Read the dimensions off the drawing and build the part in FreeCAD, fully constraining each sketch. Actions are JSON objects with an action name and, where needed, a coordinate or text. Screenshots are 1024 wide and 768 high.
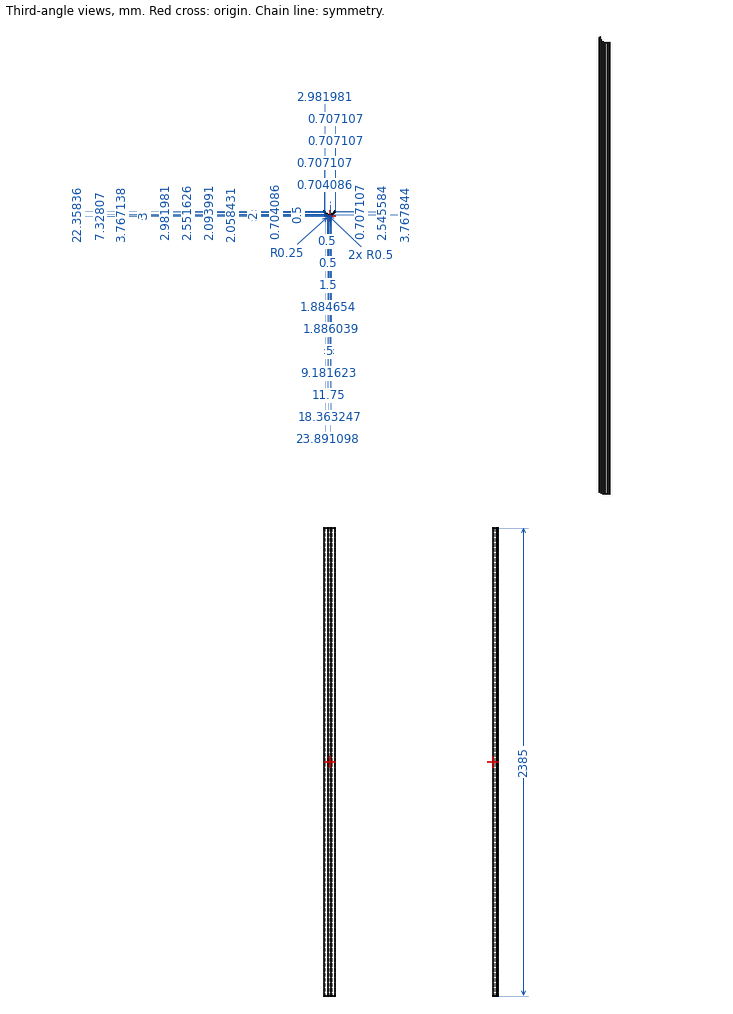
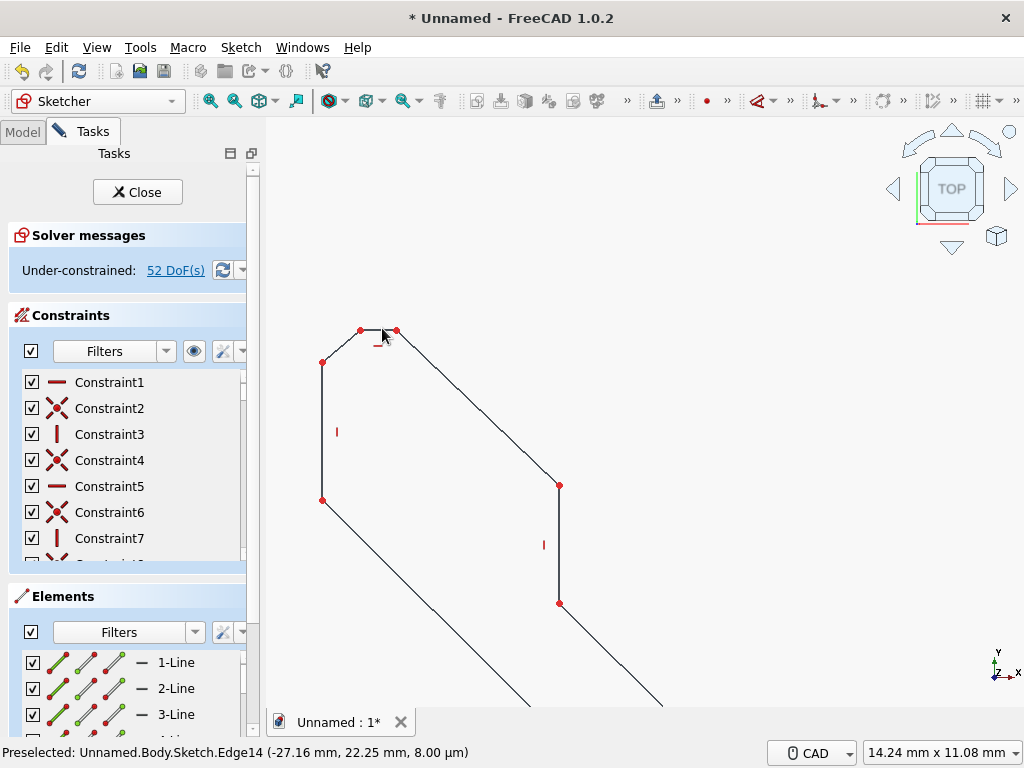
{"action": "scroll", "coordinate": [381, 333], "scroll_direction": "down", "scroll_amount": 10}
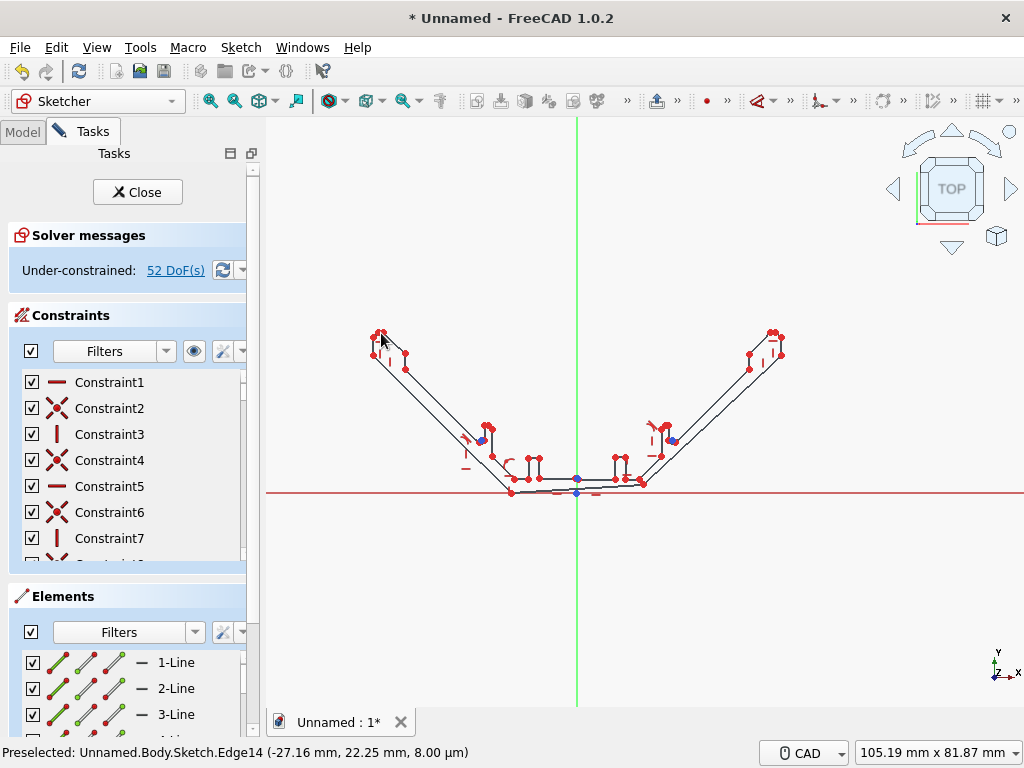
{"action": "scroll", "coordinate": [551, 491], "scroll_direction": "up", "scroll_amount": 9}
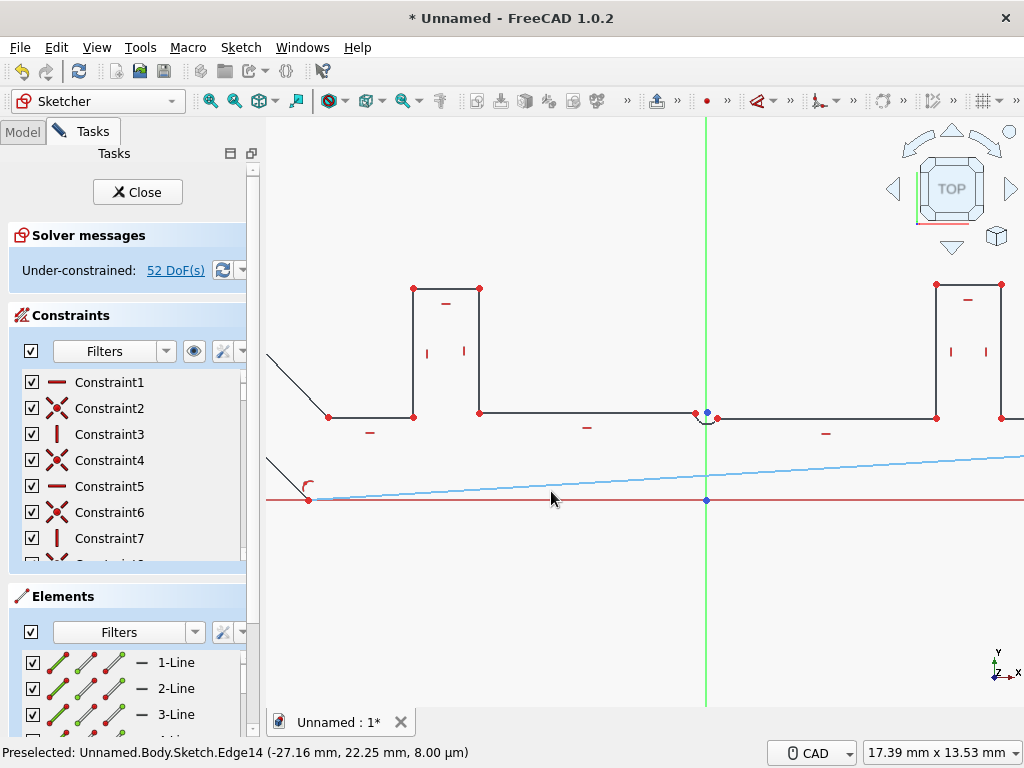
{"action": "left_click", "coordinate": [548, 485]}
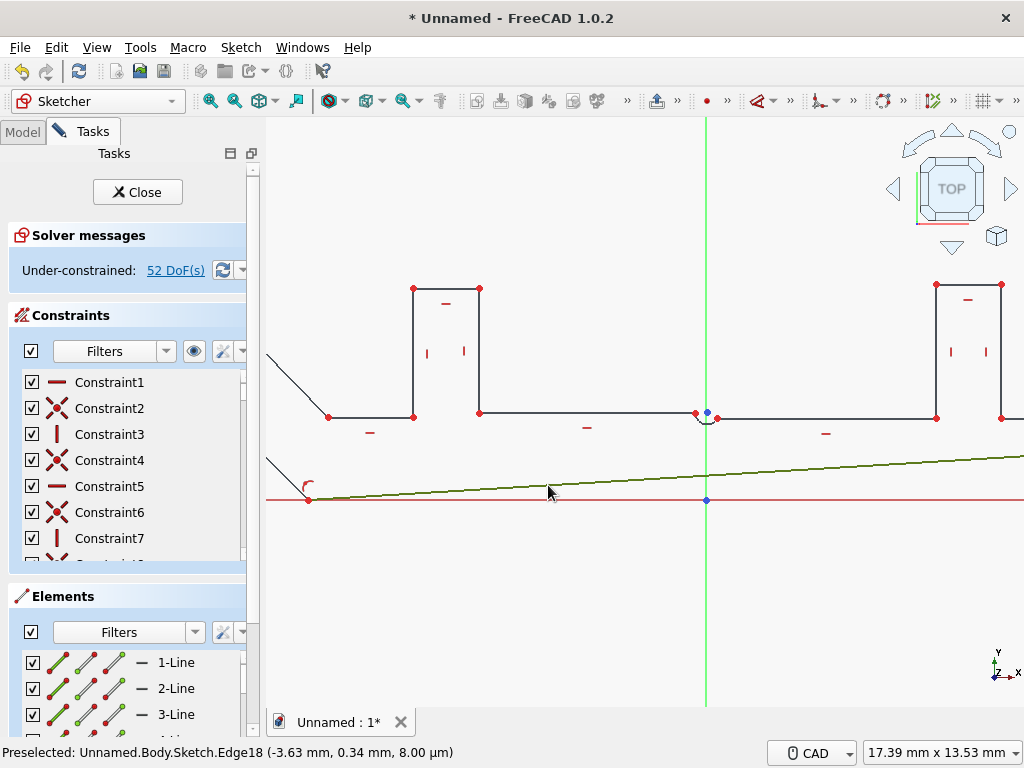
{"action": "key", "text": "h"}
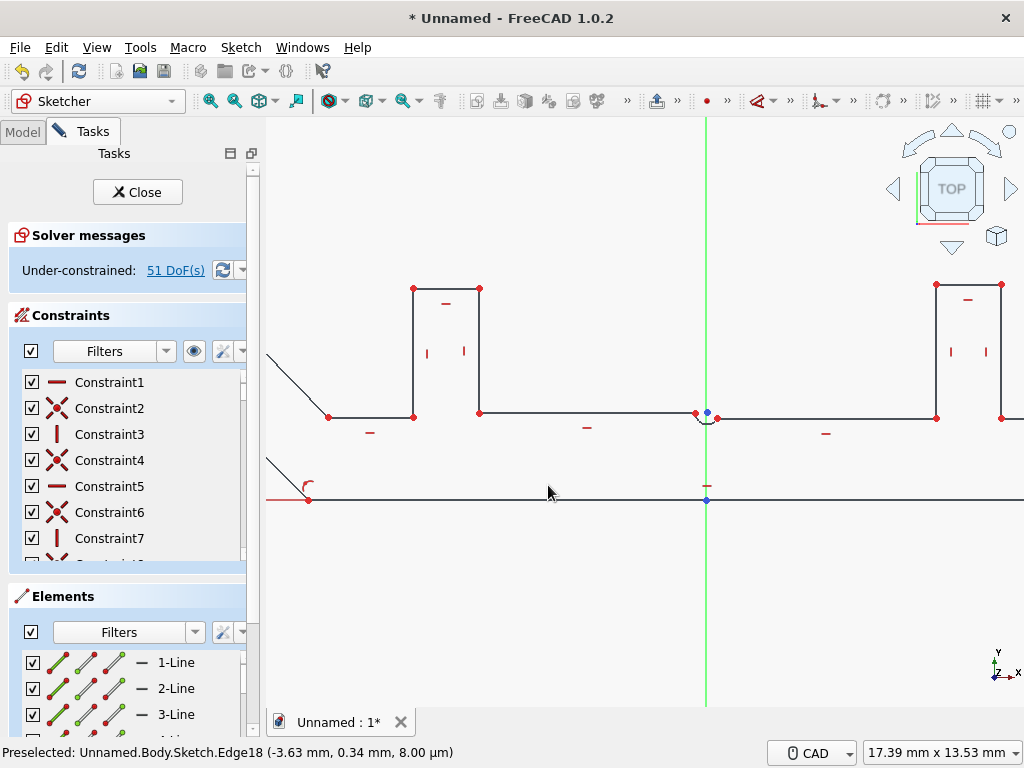
{"action": "scroll", "coordinate": [551, 491], "scroll_direction": "down", "scroll_amount": 9}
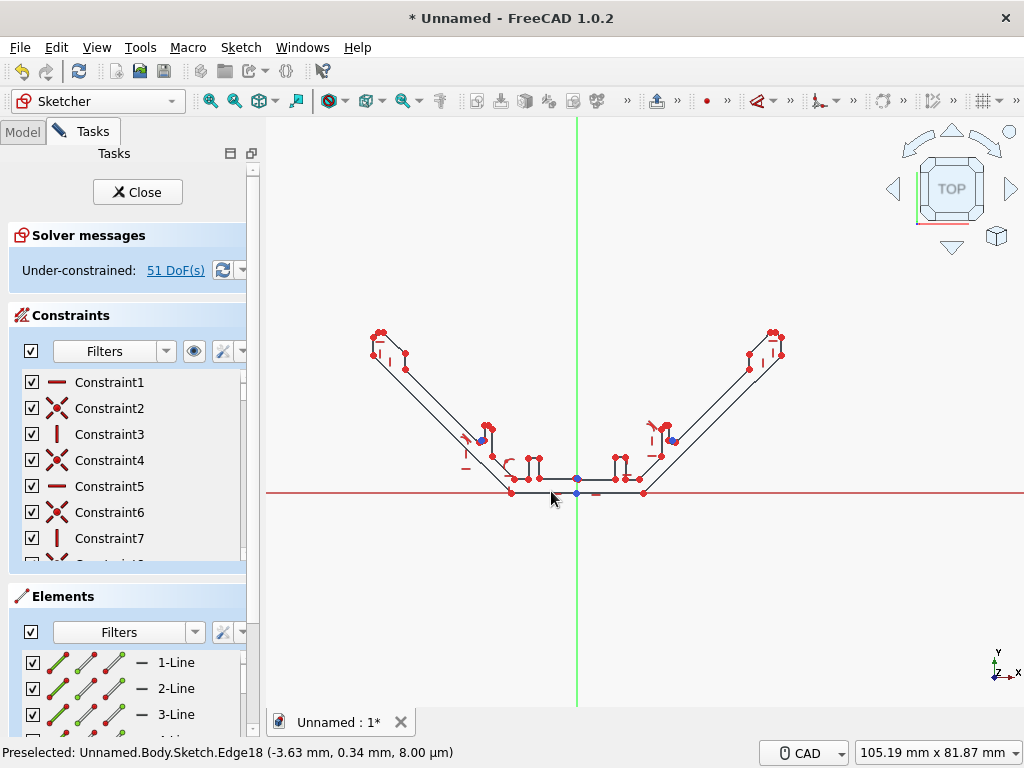
{"action": "scroll", "coordinate": [481, 444], "scroll_direction": "up", "scroll_amount": 9}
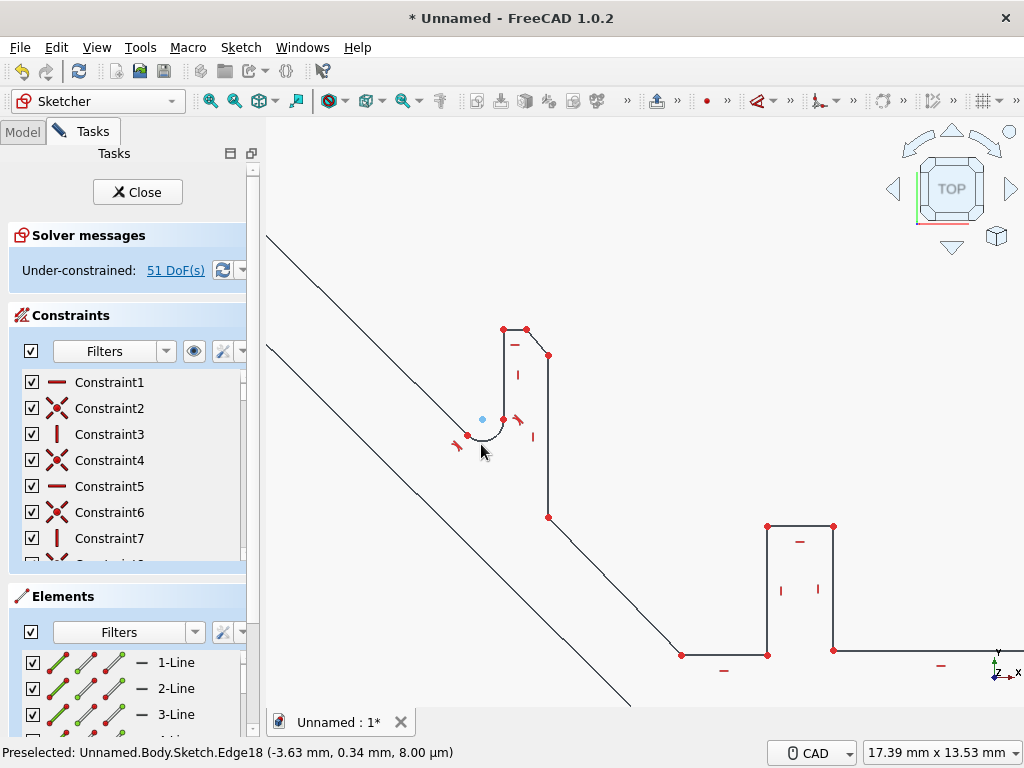
{"action": "left_click", "coordinate": [481, 441]}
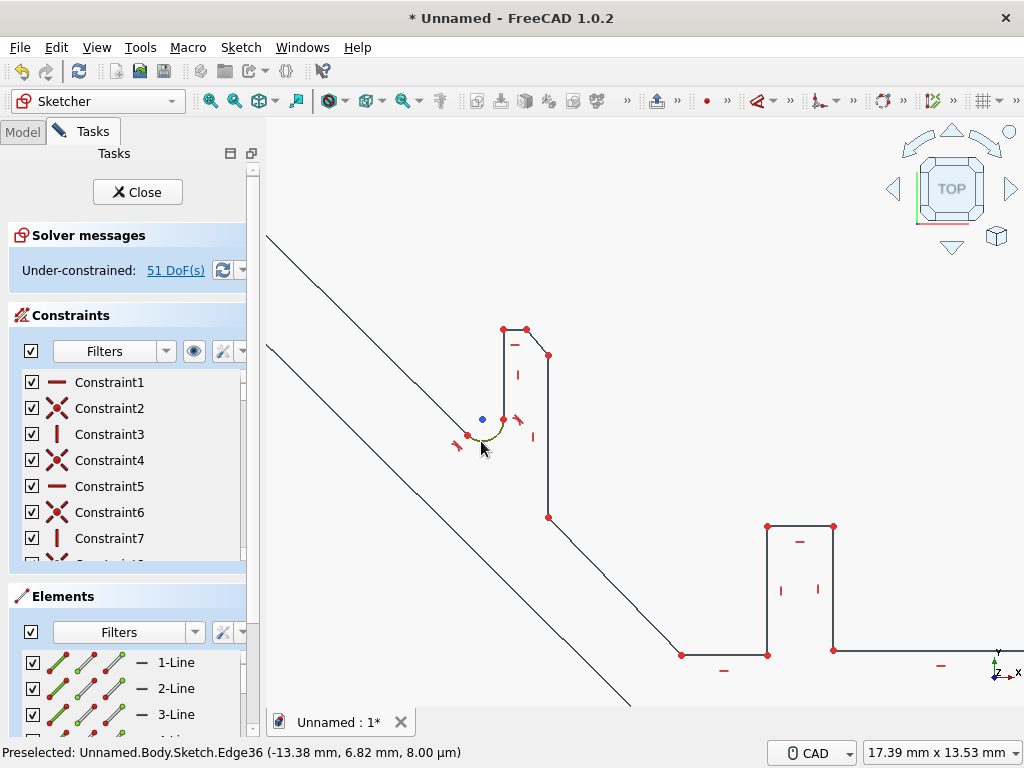
{"action": "scroll", "coordinate": [481, 444], "scroll_direction": "down", "scroll_amount": 9}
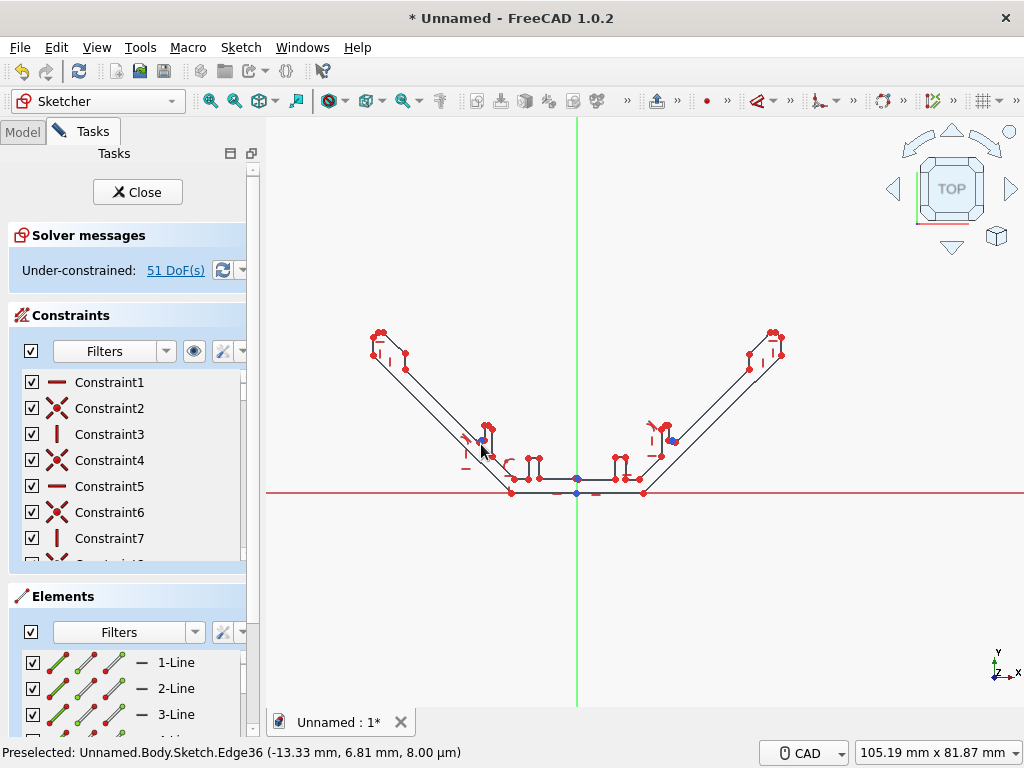
{"action": "scroll", "coordinate": [670, 443], "scroll_direction": "up", "scroll_amount": 9}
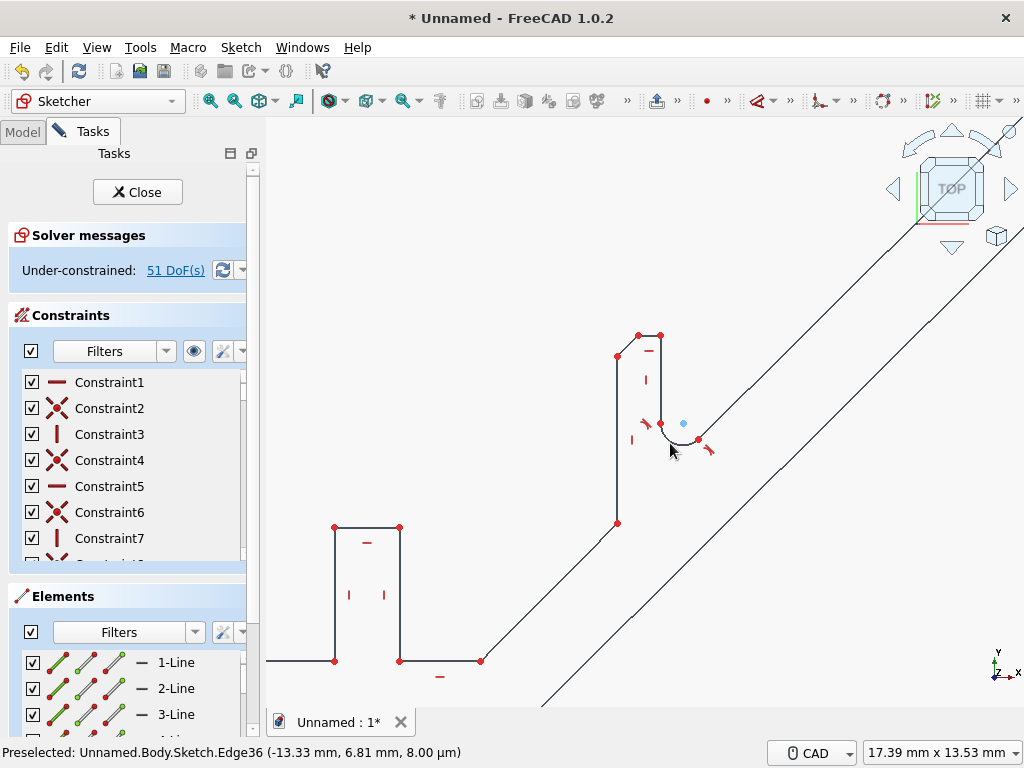
{"action": "left_click", "coordinate": [666, 438]}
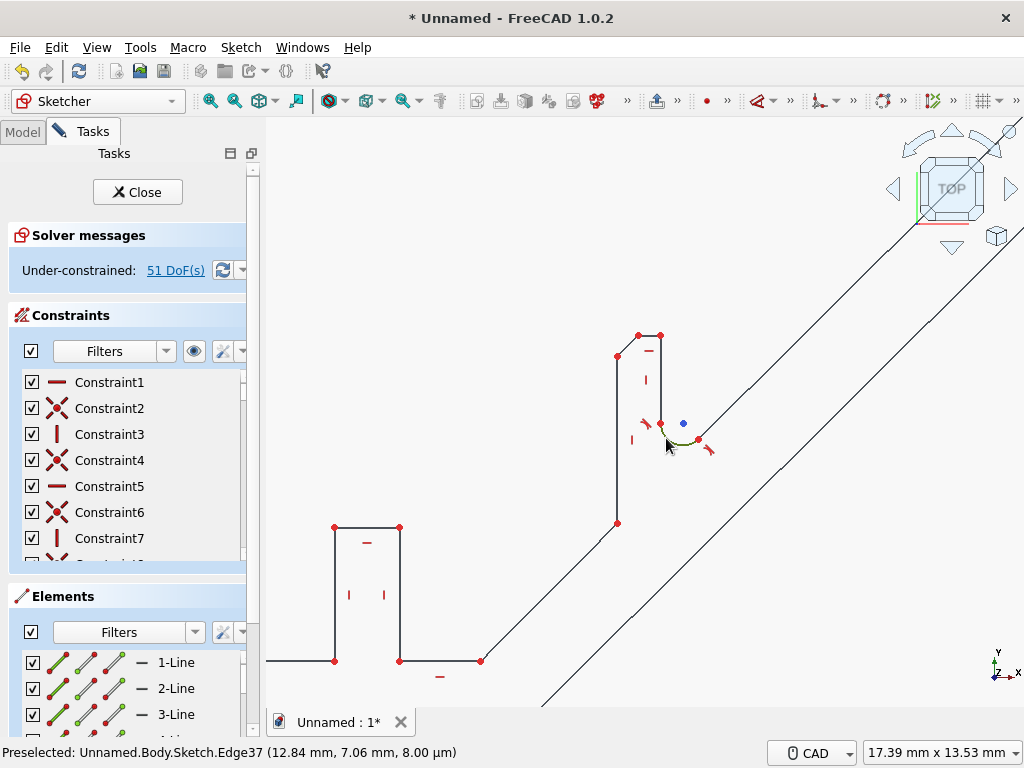
{"action": "key", "text": "e"}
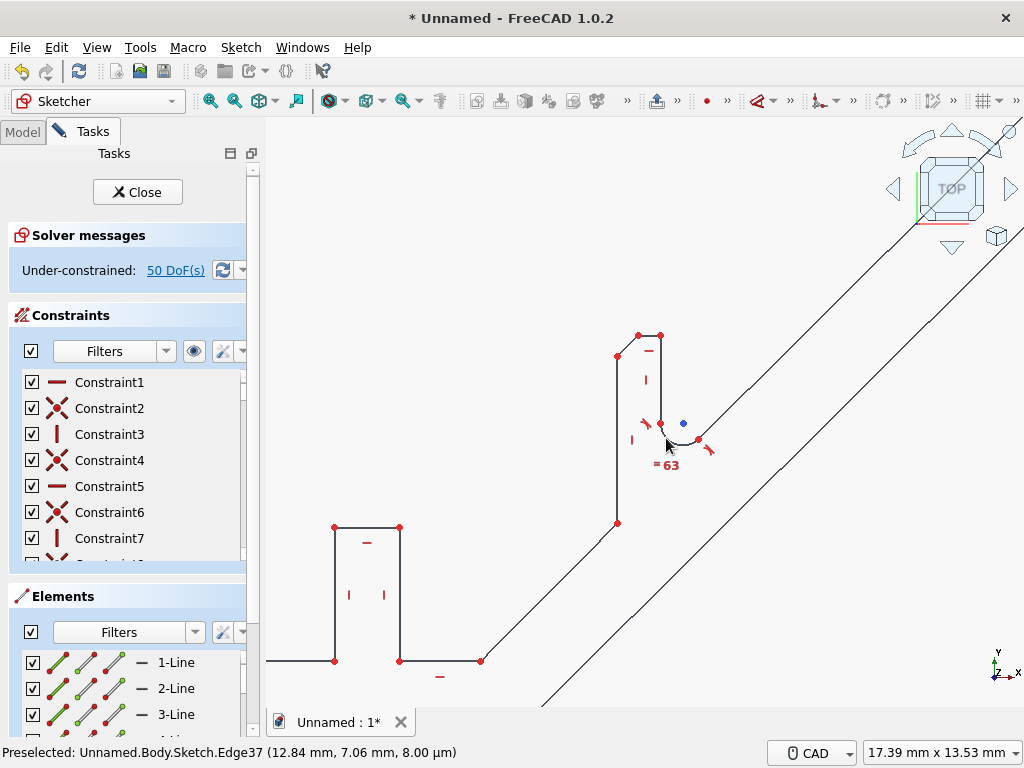
{"action": "scroll", "coordinate": [670, 443], "scroll_direction": "down", "scroll_amount": 9}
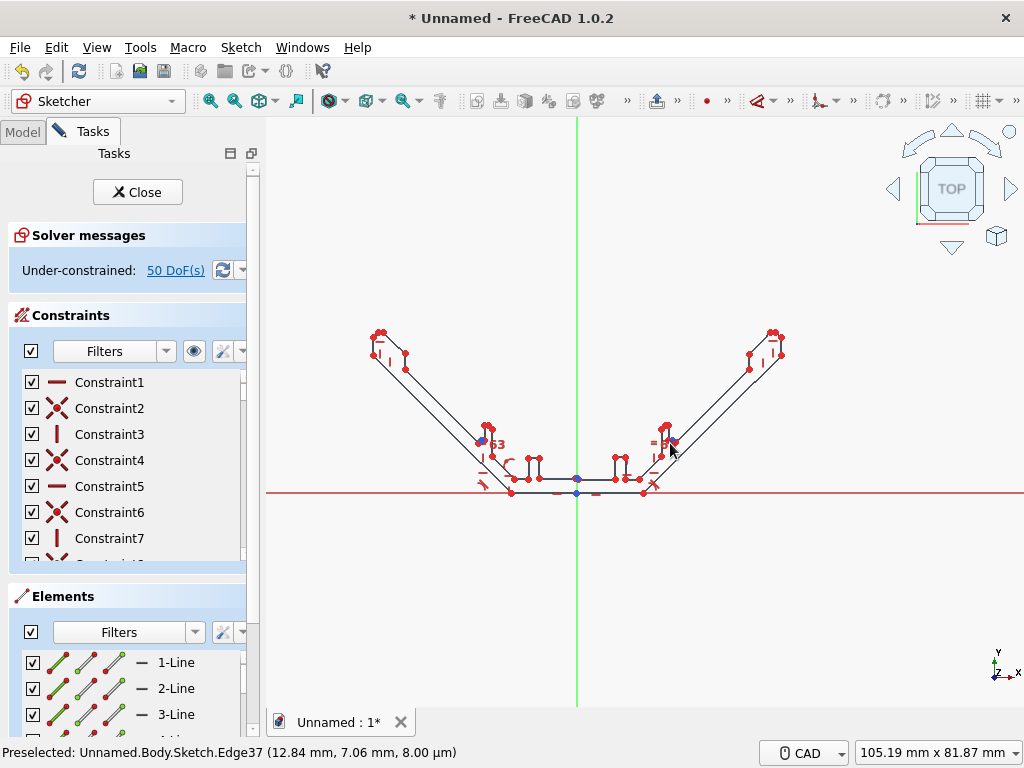
{"action": "scroll", "coordinate": [577, 479], "scroll_direction": "up", "scroll_amount": 10}